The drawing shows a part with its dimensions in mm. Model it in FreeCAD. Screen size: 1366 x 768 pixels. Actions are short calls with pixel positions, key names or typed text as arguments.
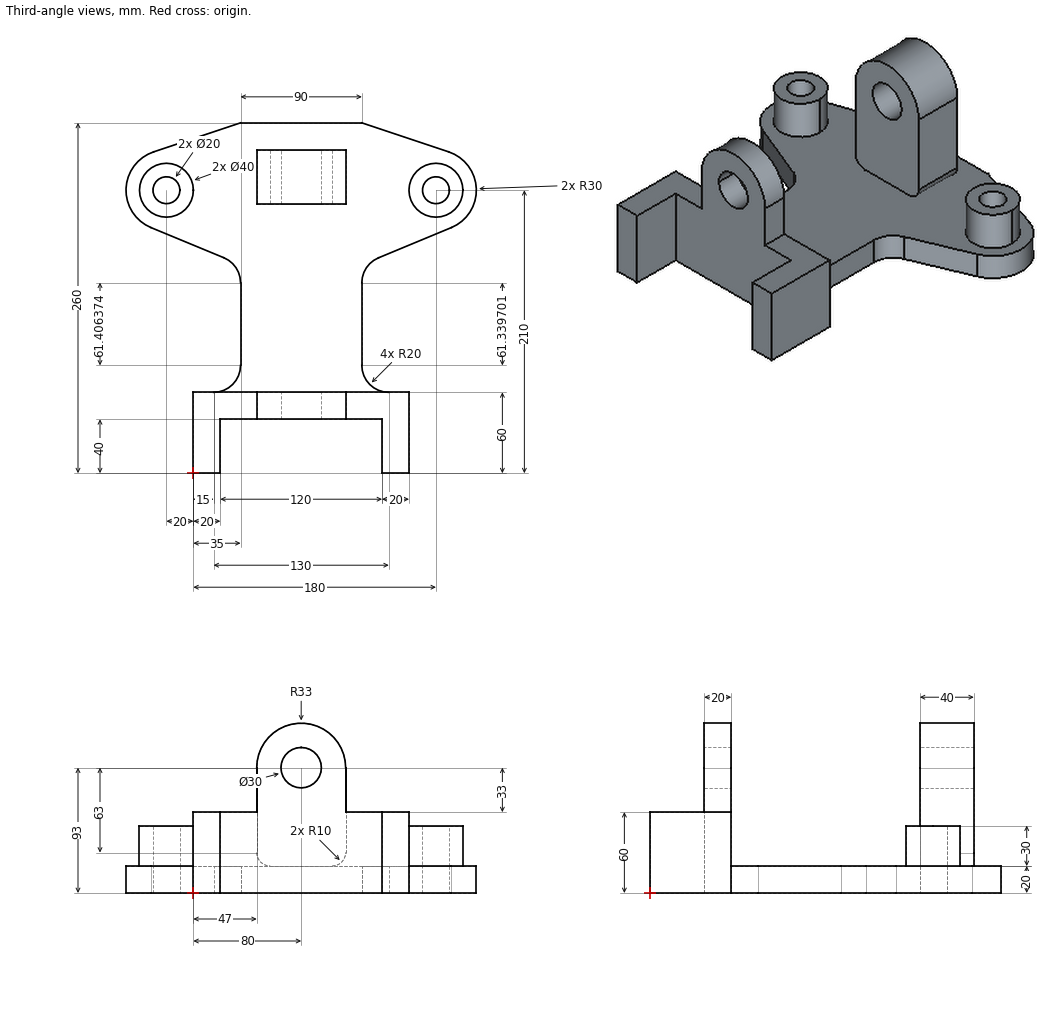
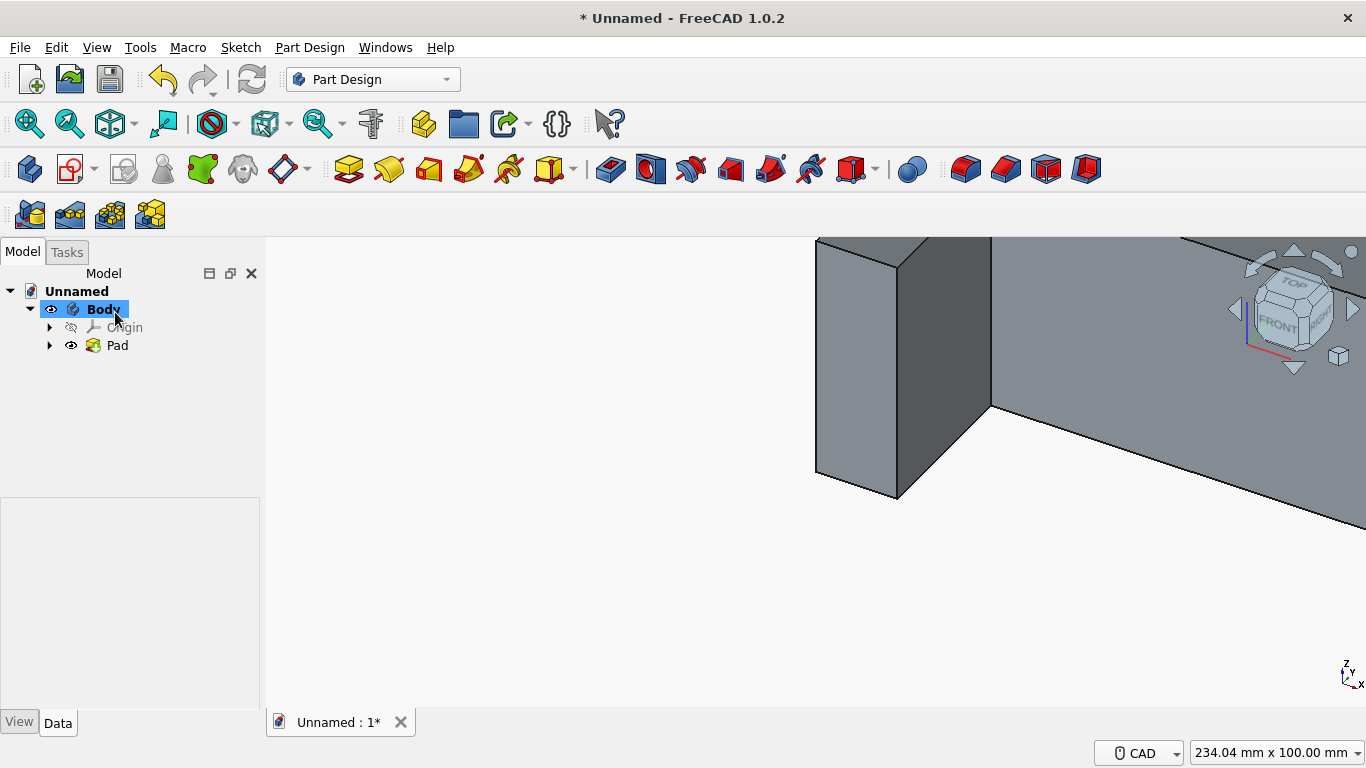
key(v)
key(f)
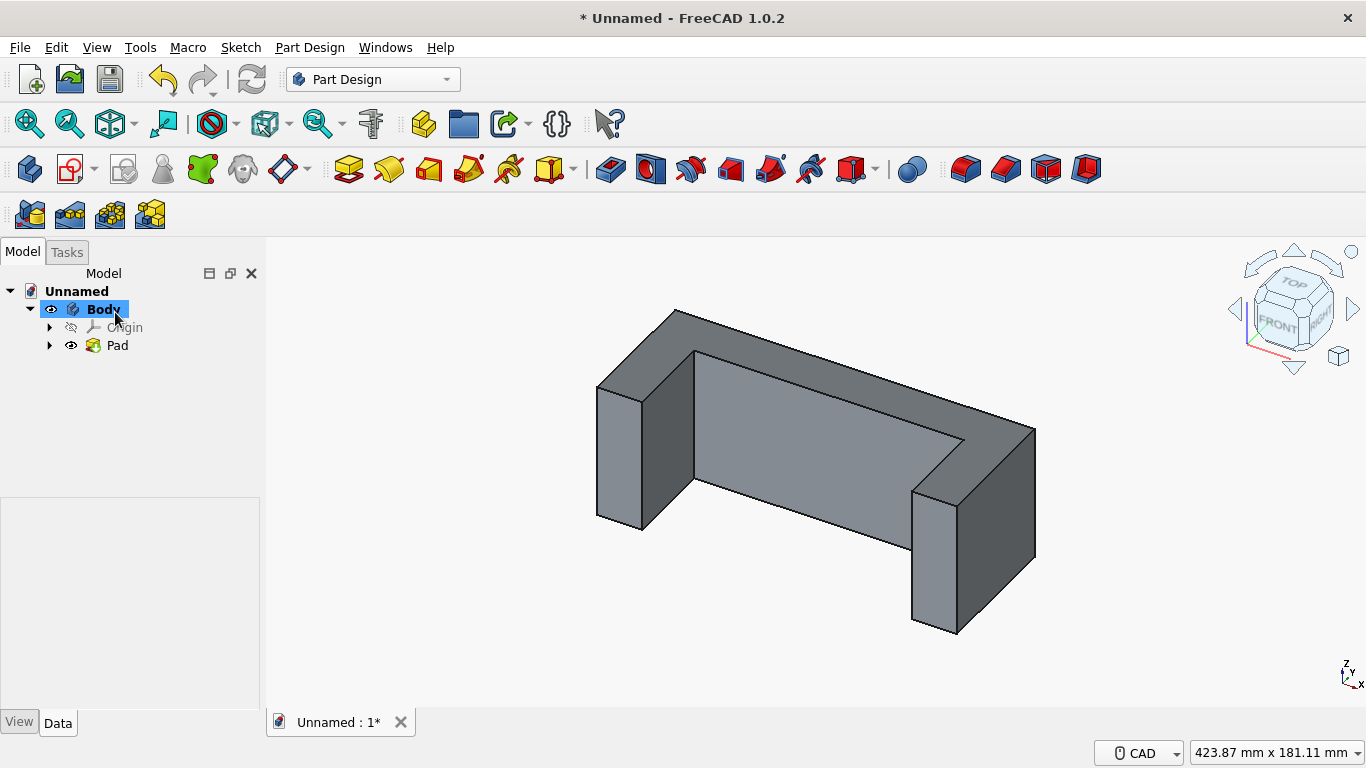
key(4)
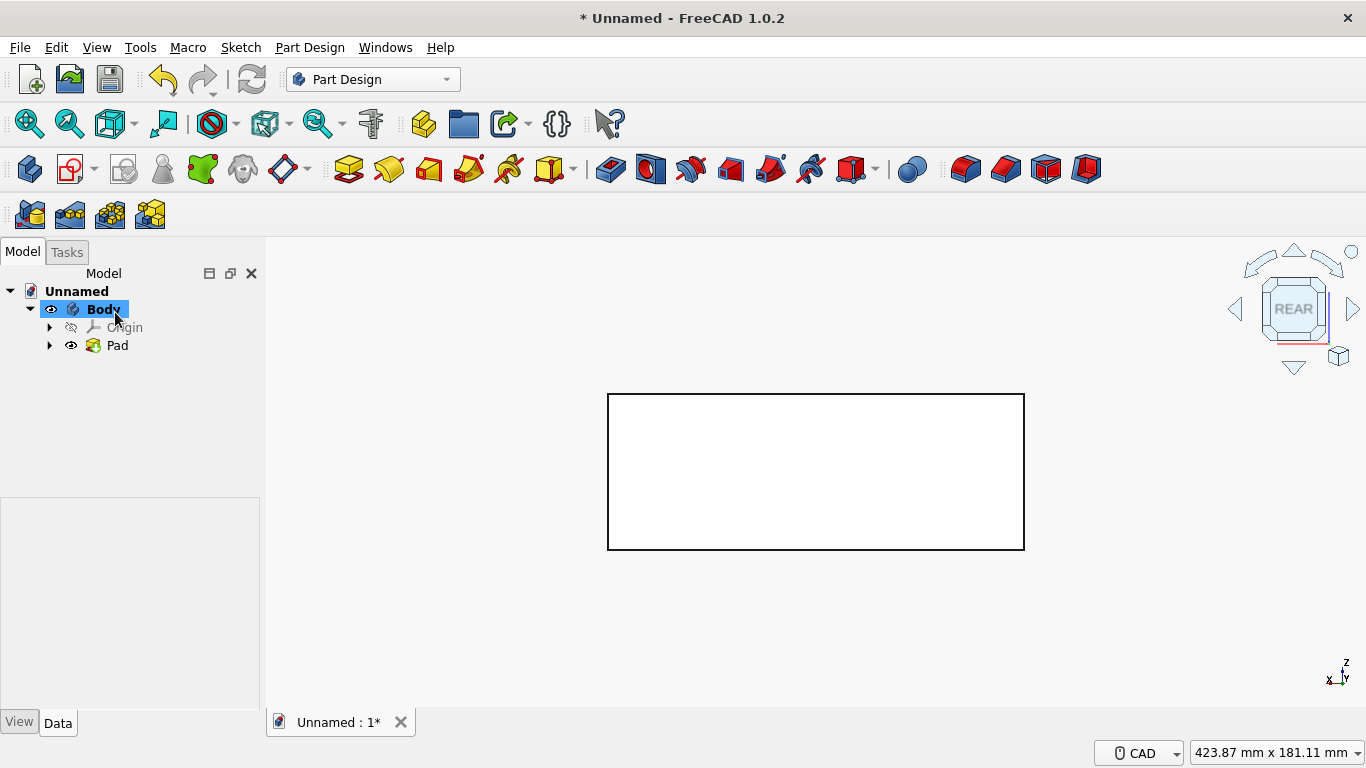
key(v)
key(f)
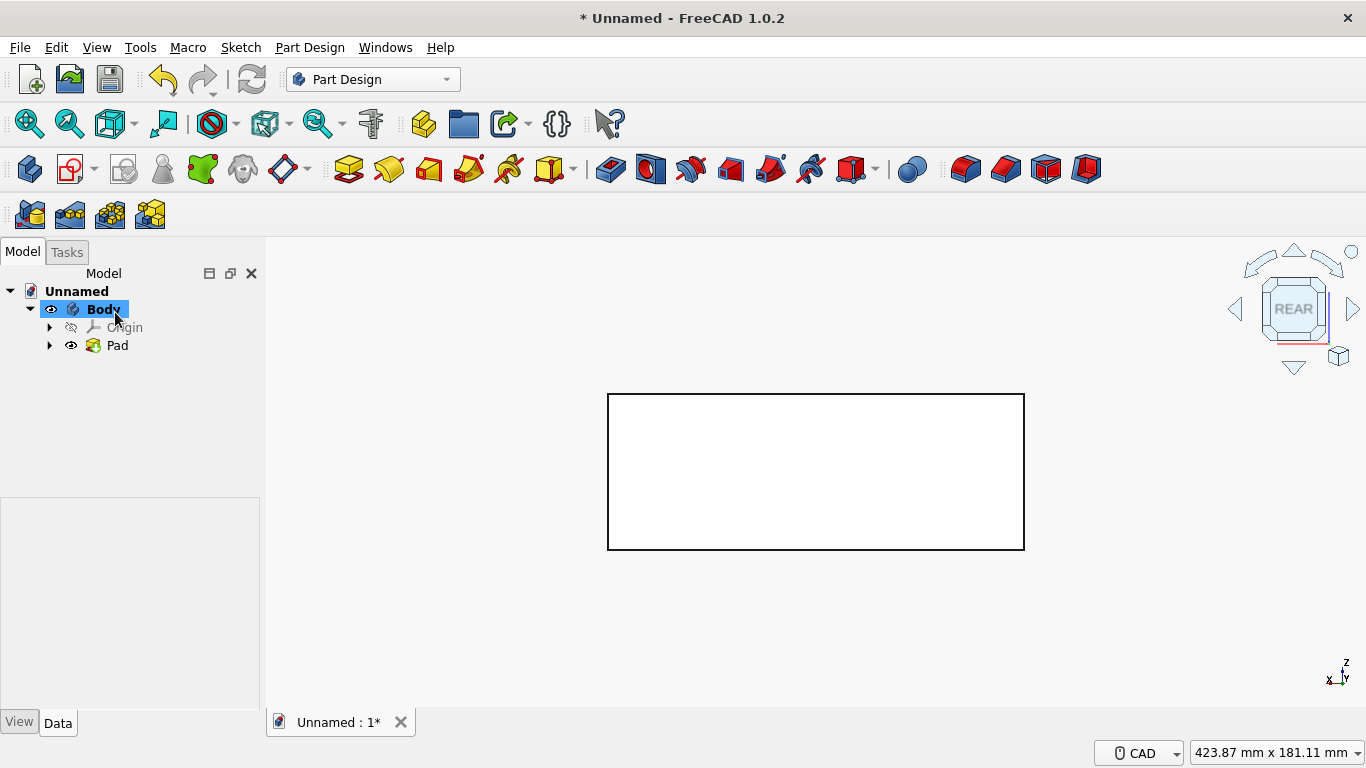
click(697, 471)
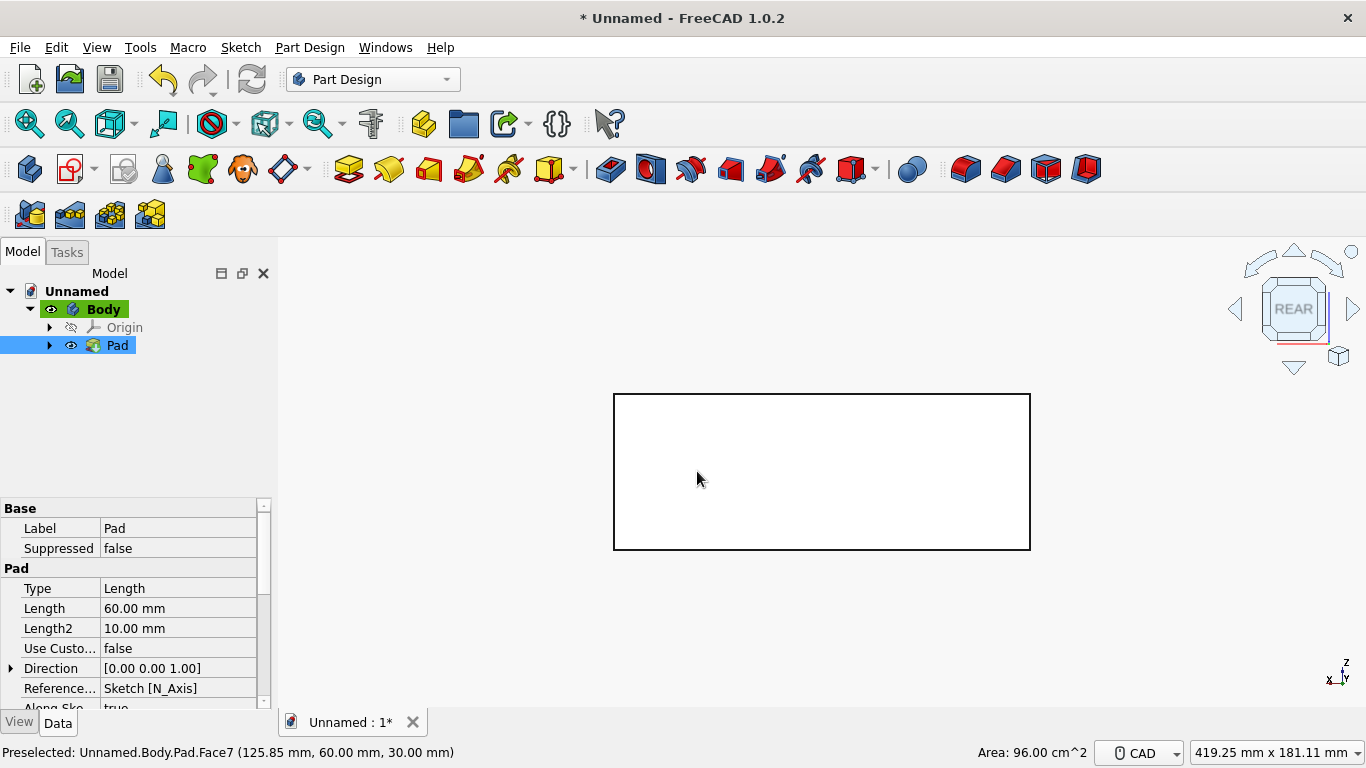
click(70, 170)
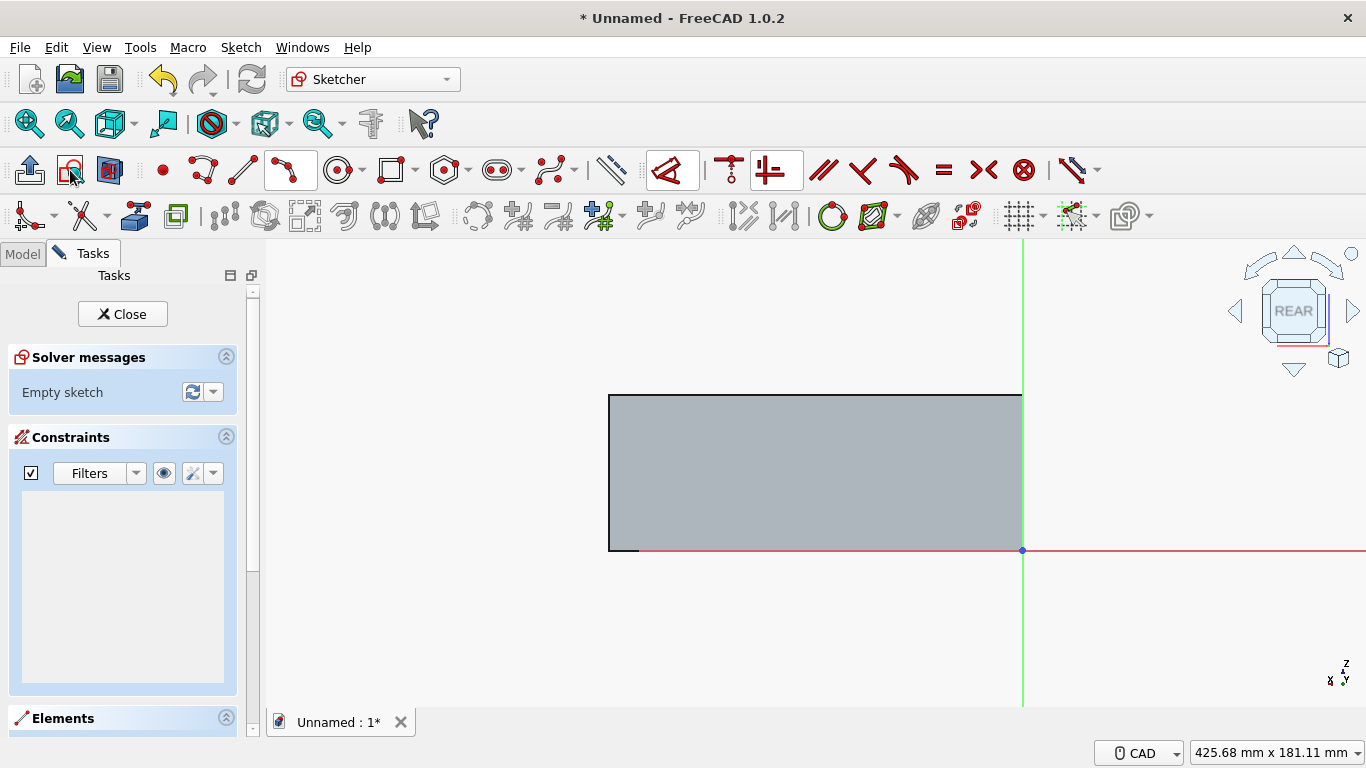
scroll(294, 679, down, 1)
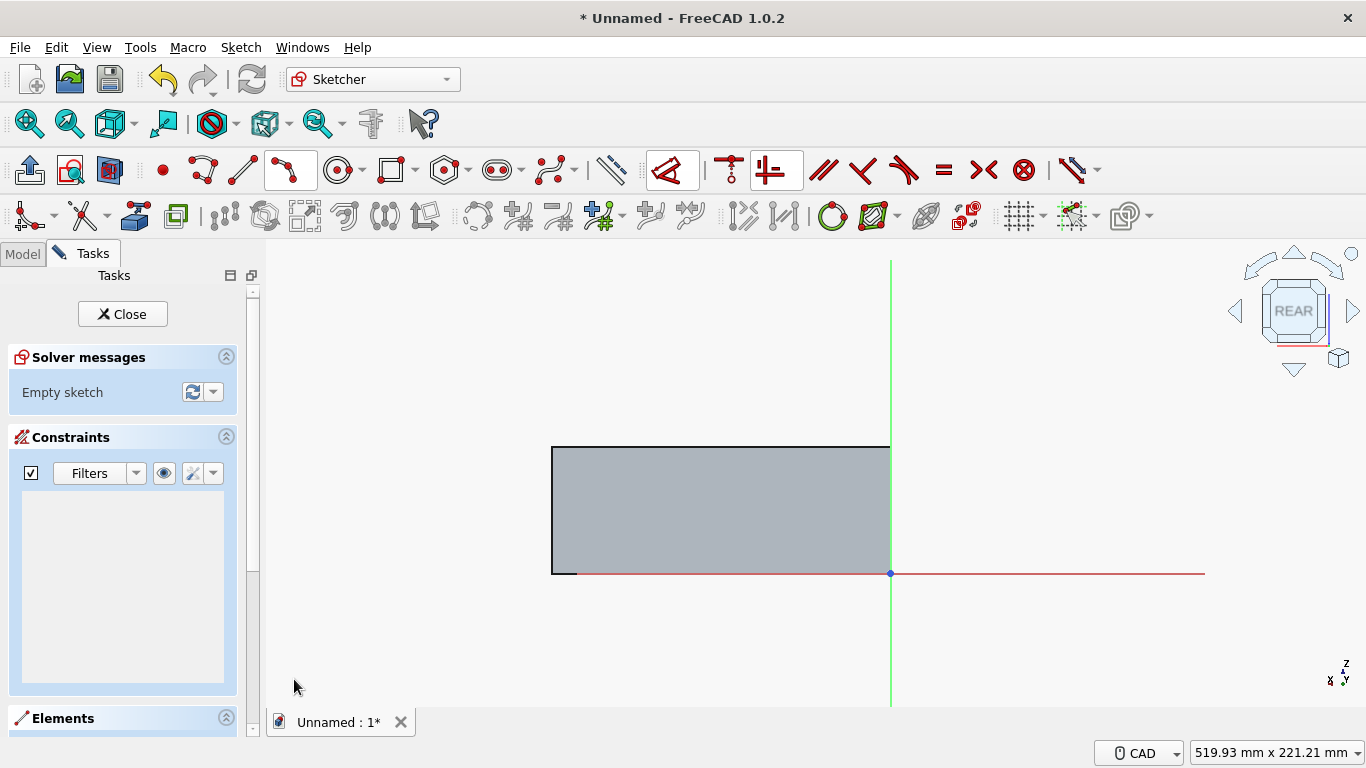
click(204, 170)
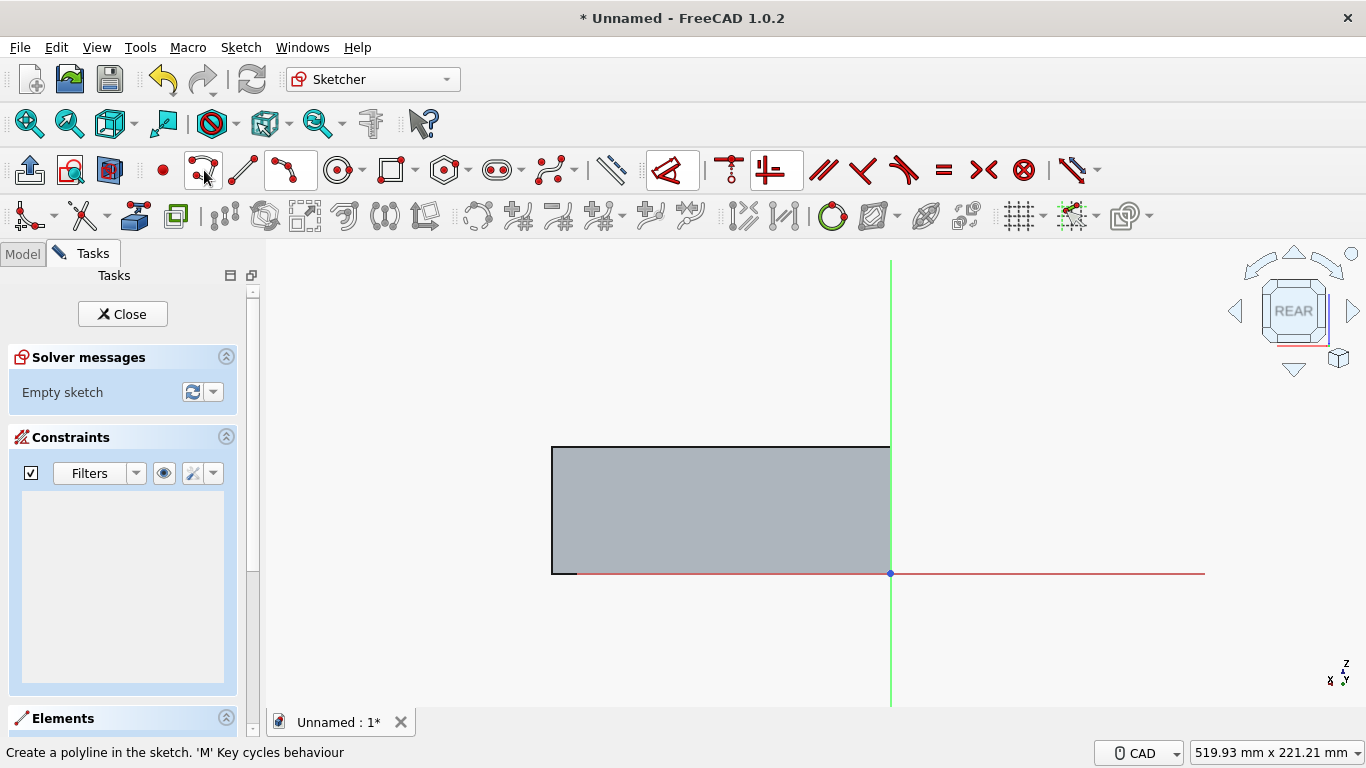
click(652, 377)
click(652, 447)
click(791, 447)
click(791, 377)
right_click(791, 377)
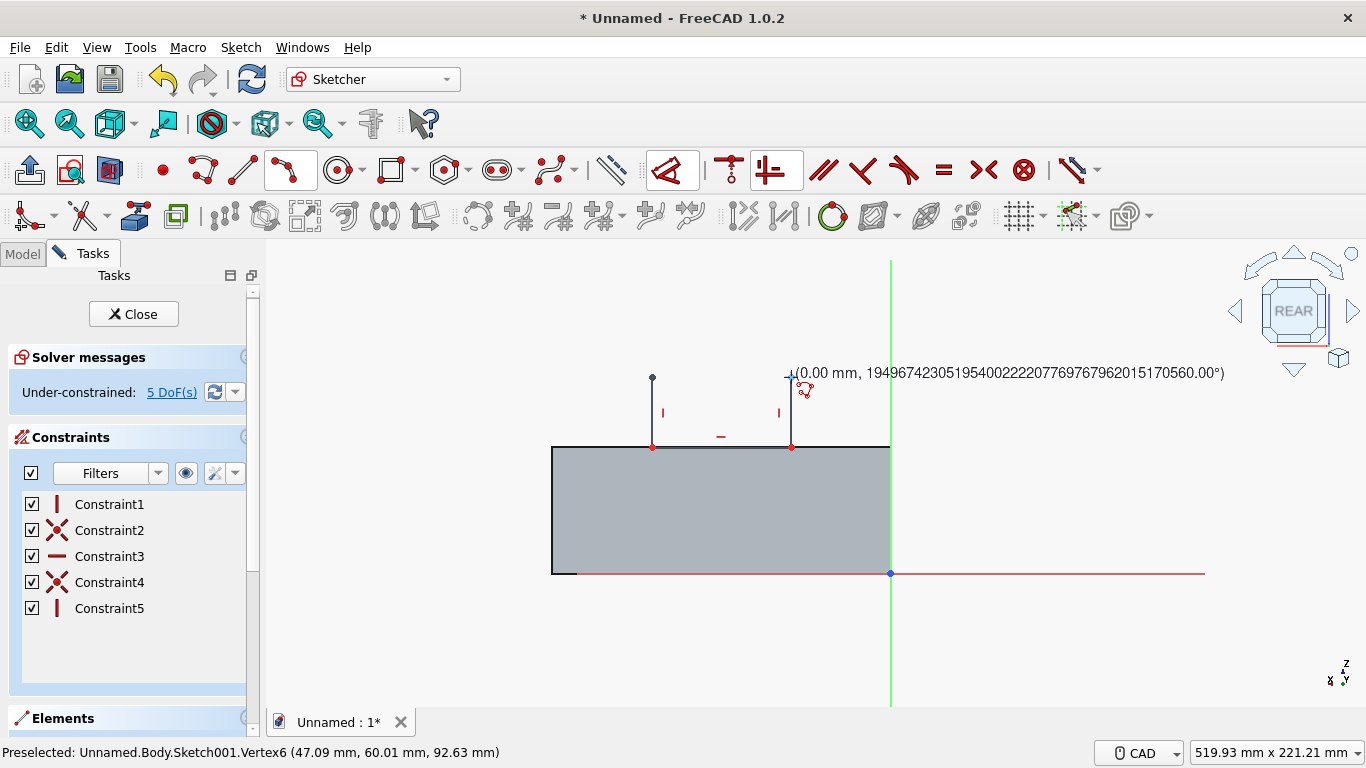
click(284, 170)